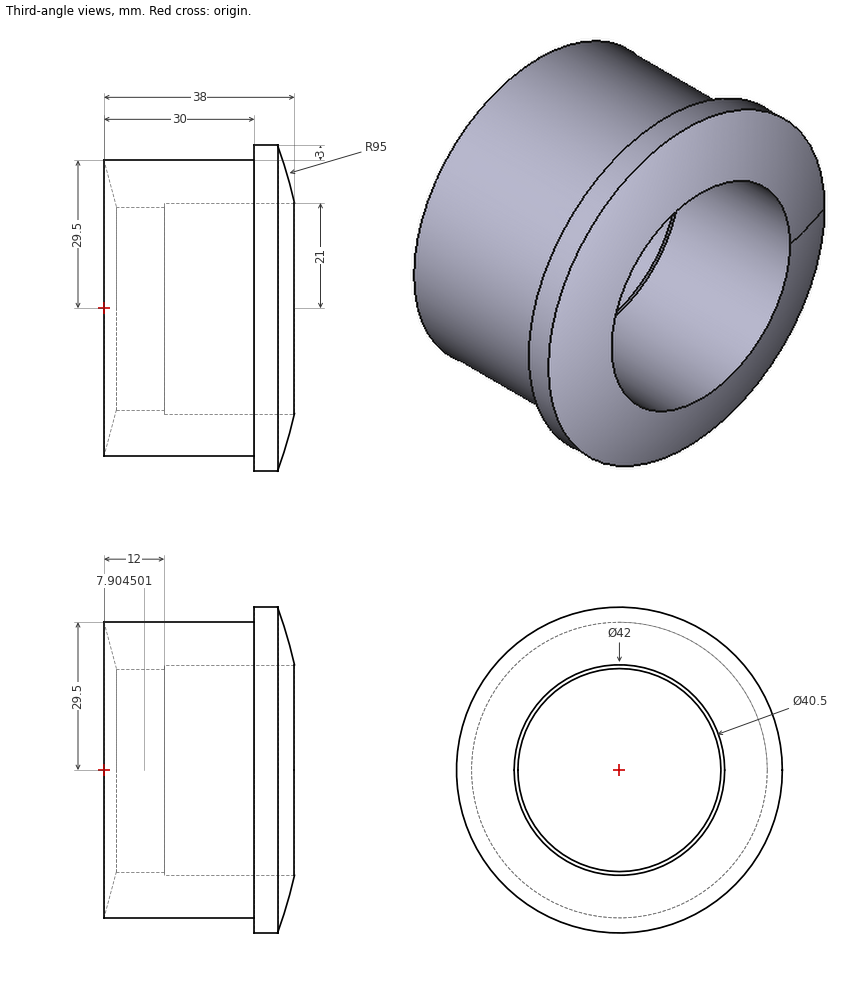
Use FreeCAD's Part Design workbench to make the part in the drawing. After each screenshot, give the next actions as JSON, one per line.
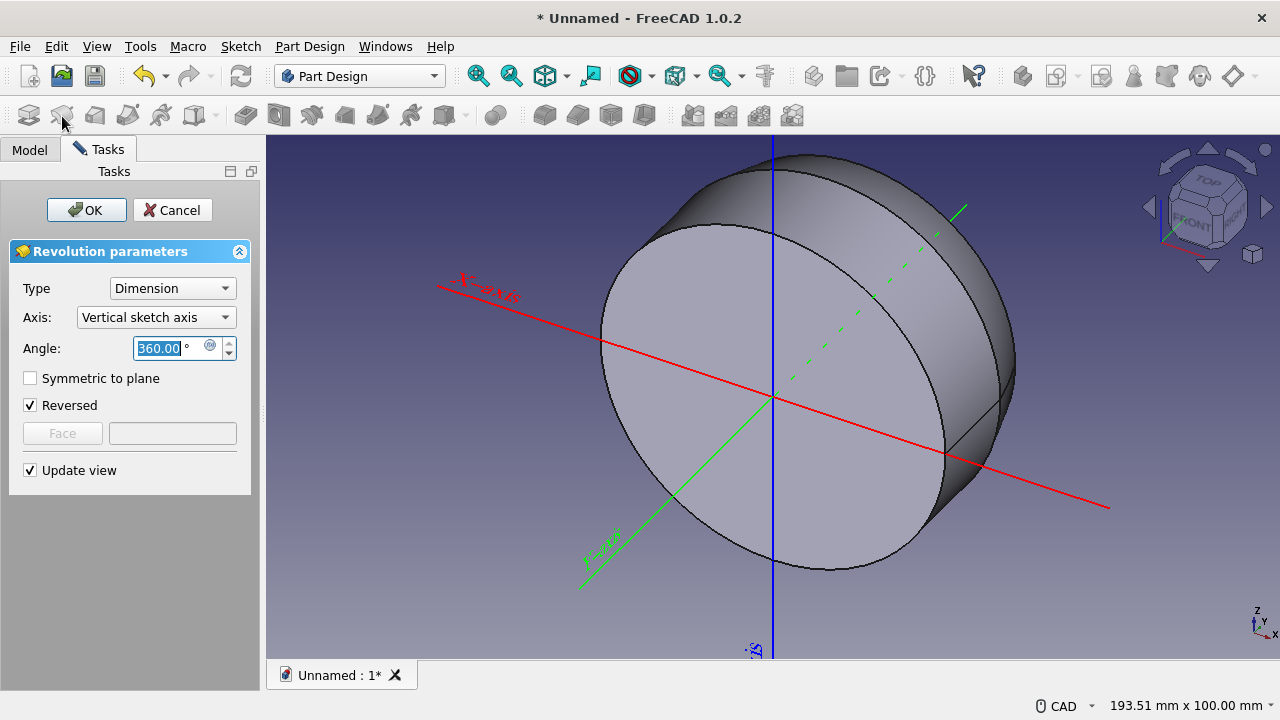
{"action": "left_click", "coordinate": [157, 318]}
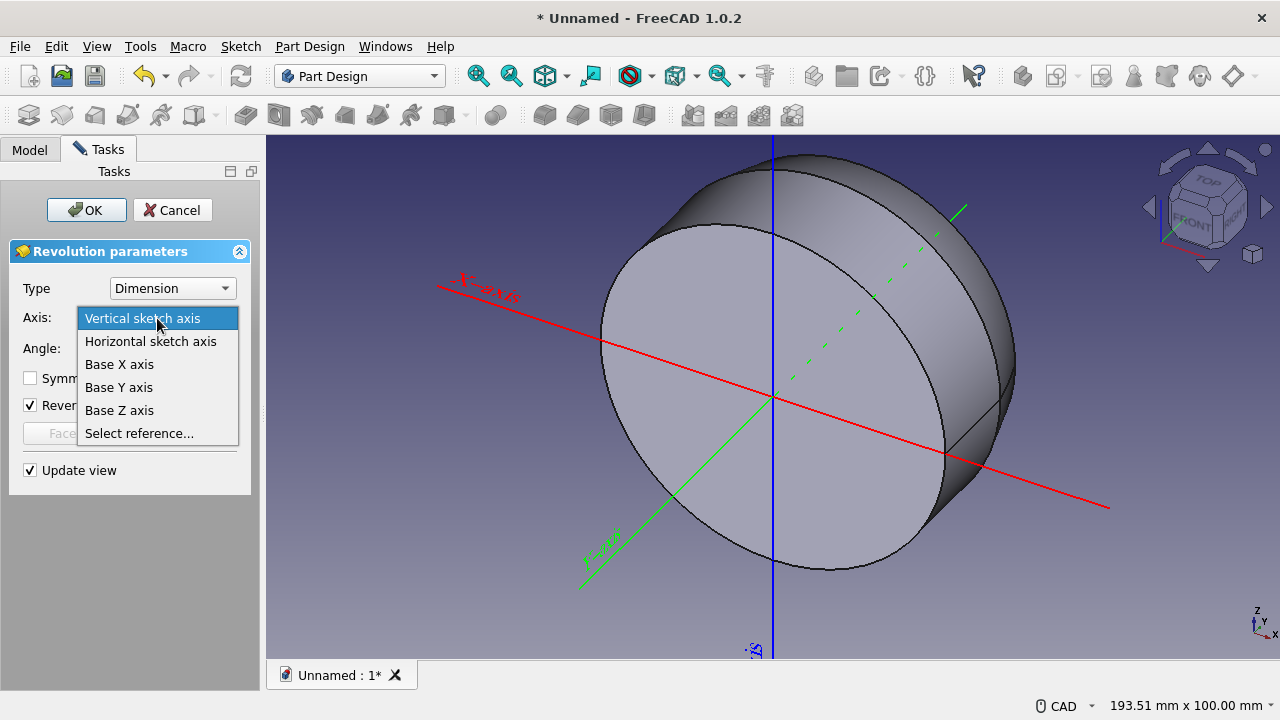
{"action": "left_click", "coordinate": [156, 342]}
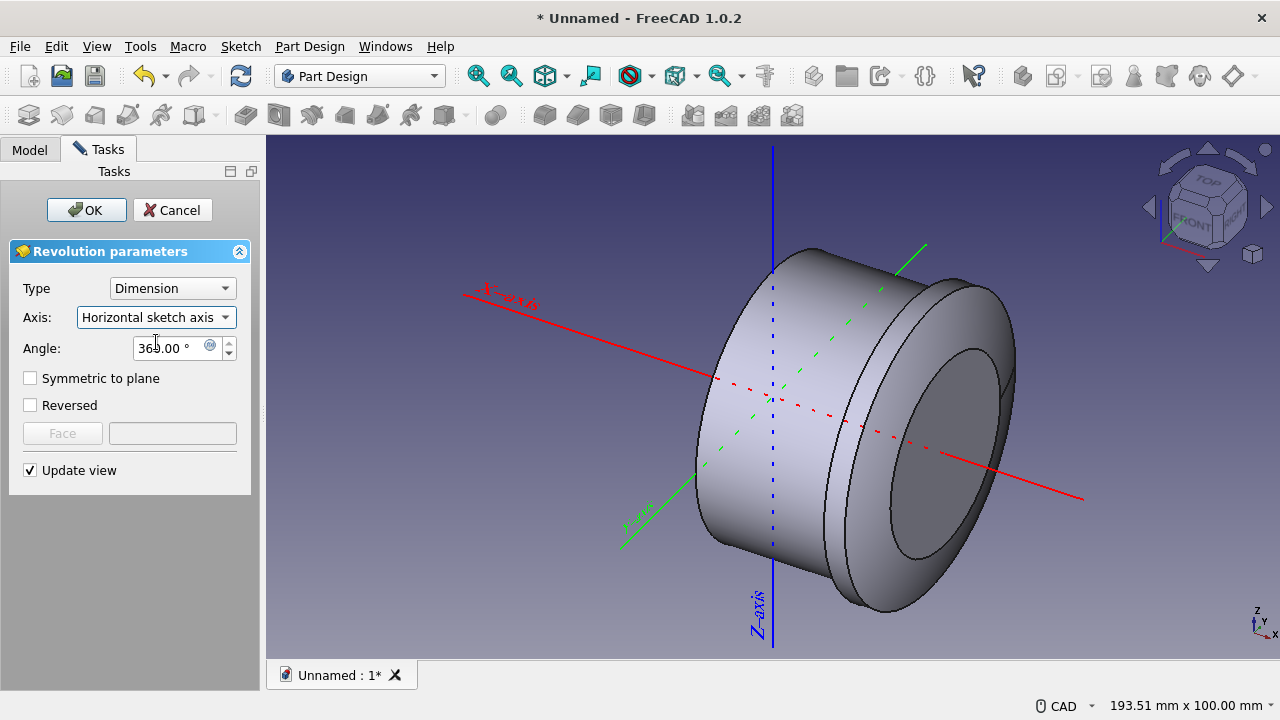
{"action": "left_click", "coordinate": [87, 210]}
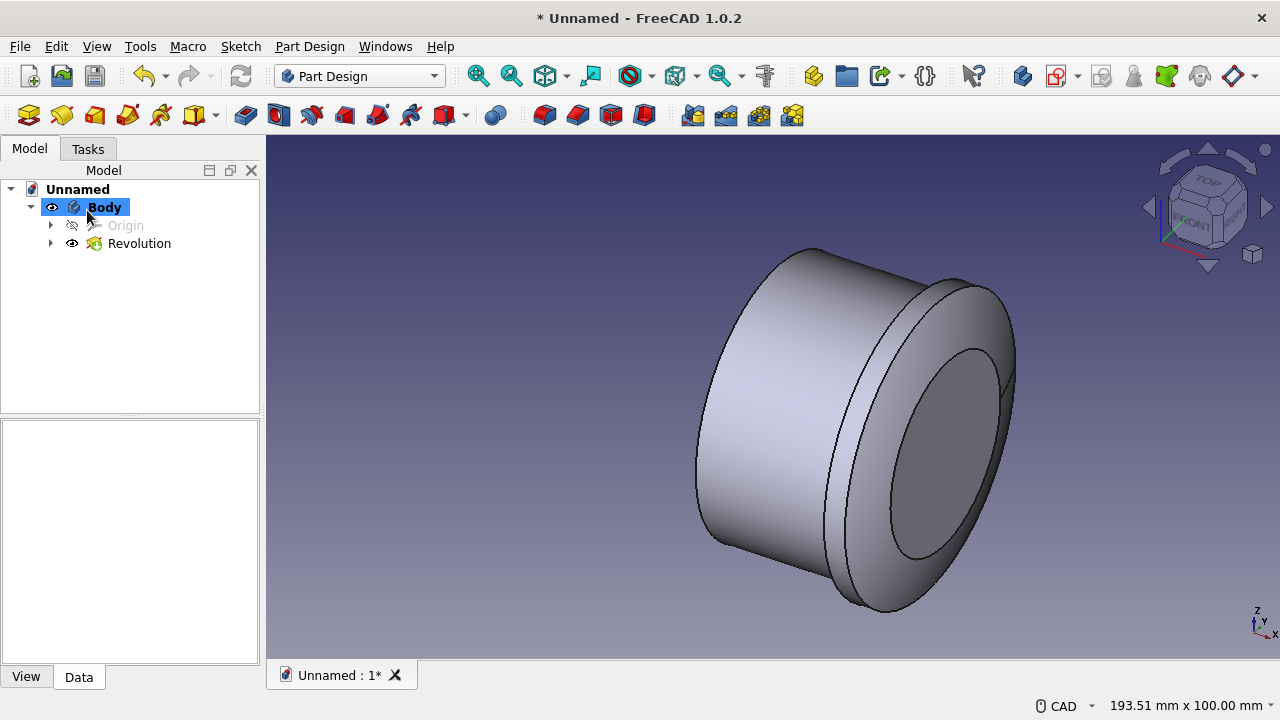
{"action": "left_click", "coordinate": [479, 76]}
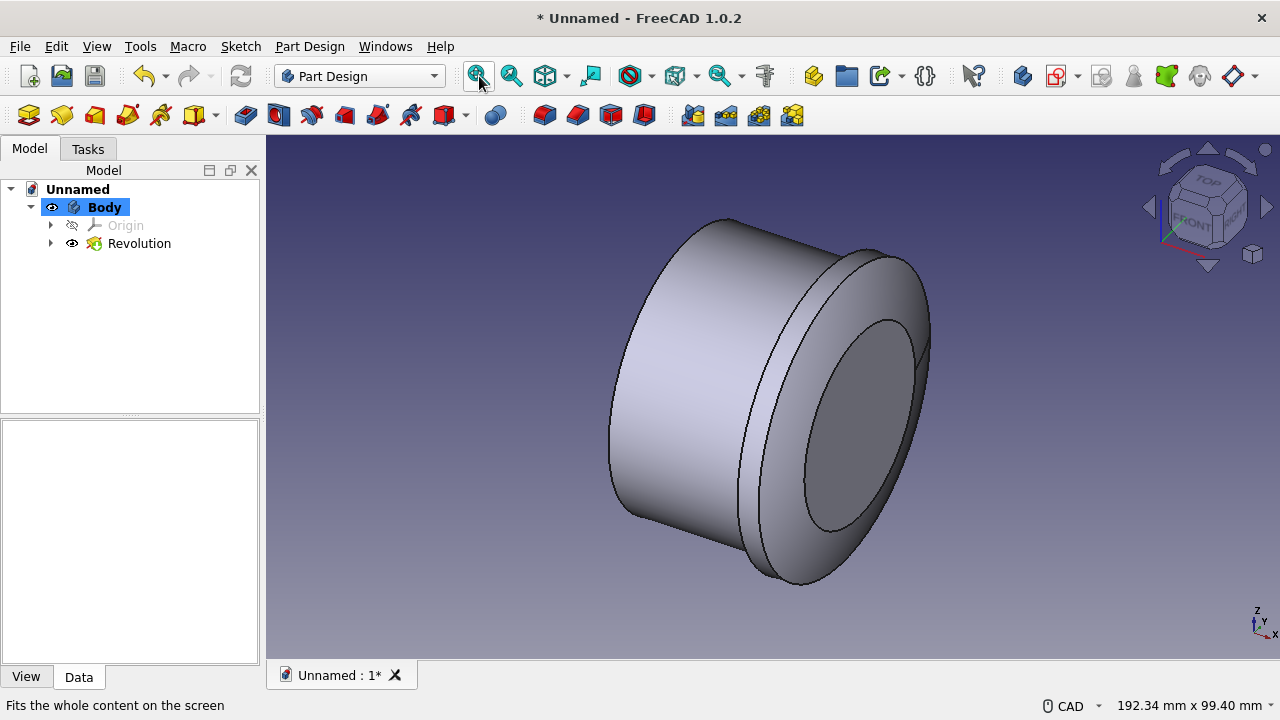
{"action": "key", "text": "6"}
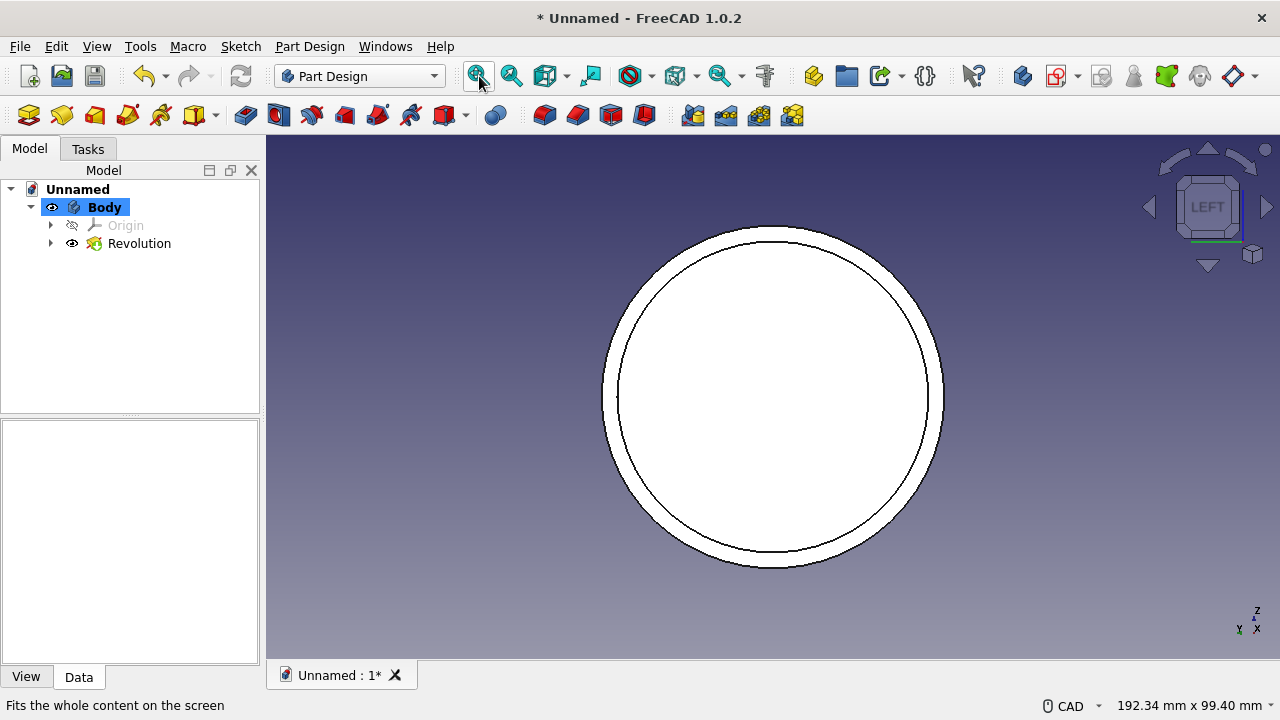
{"action": "left_click", "coordinate": [773, 396]}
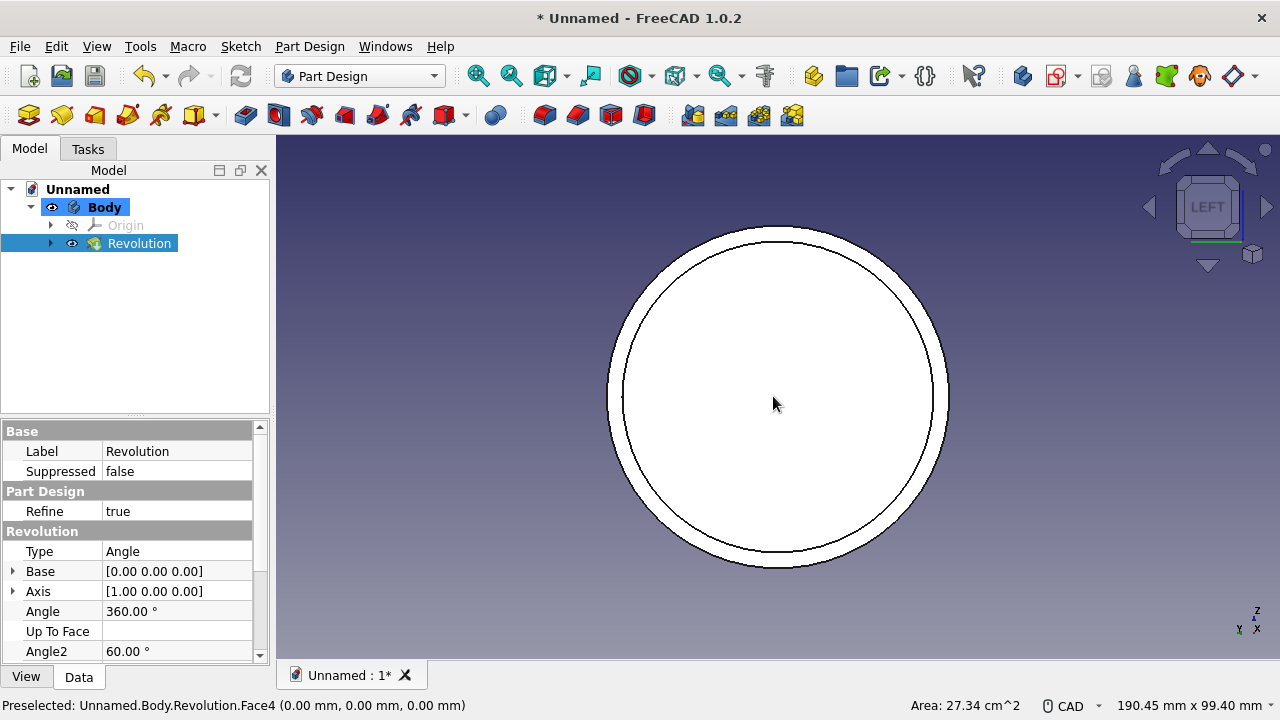
{"action": "left_click", "coordinate": [1056, 76]}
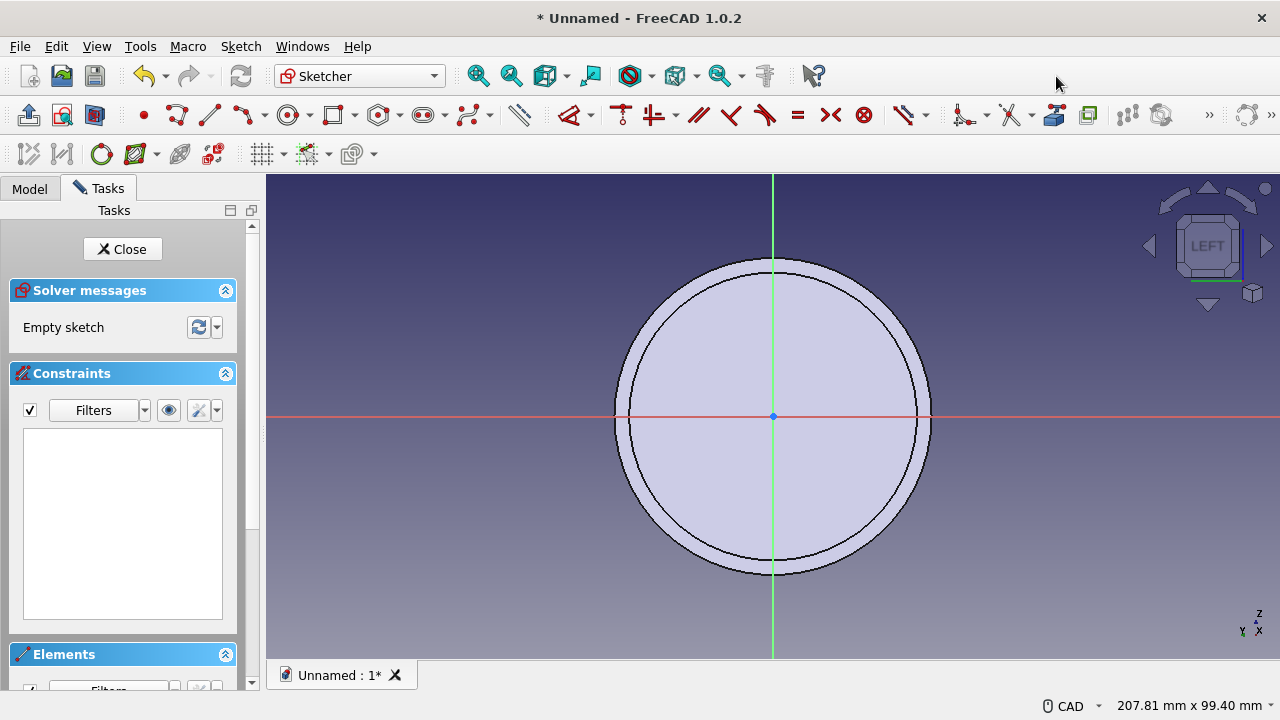
{"action": "scroll", "coordinate": [912, 416], "scroll_direction": "up", "scroll_amount": 2}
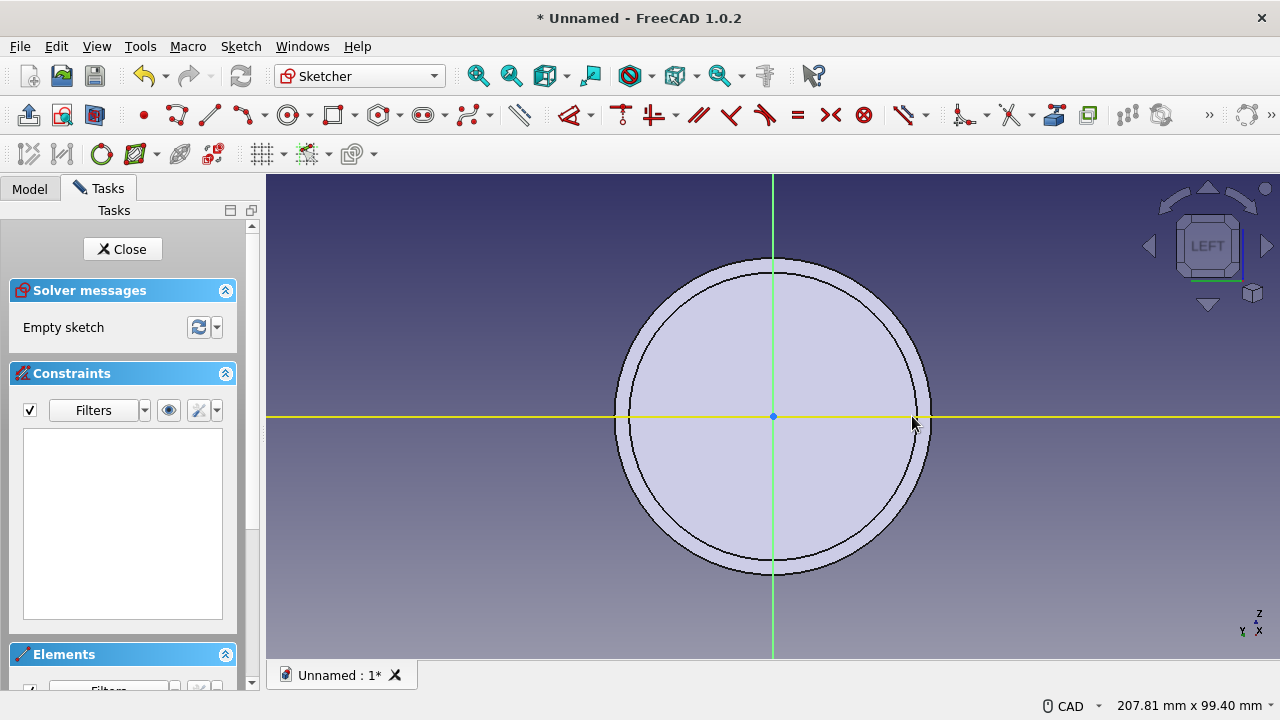
{"action": "left_click", "coordinate": [288, 116]}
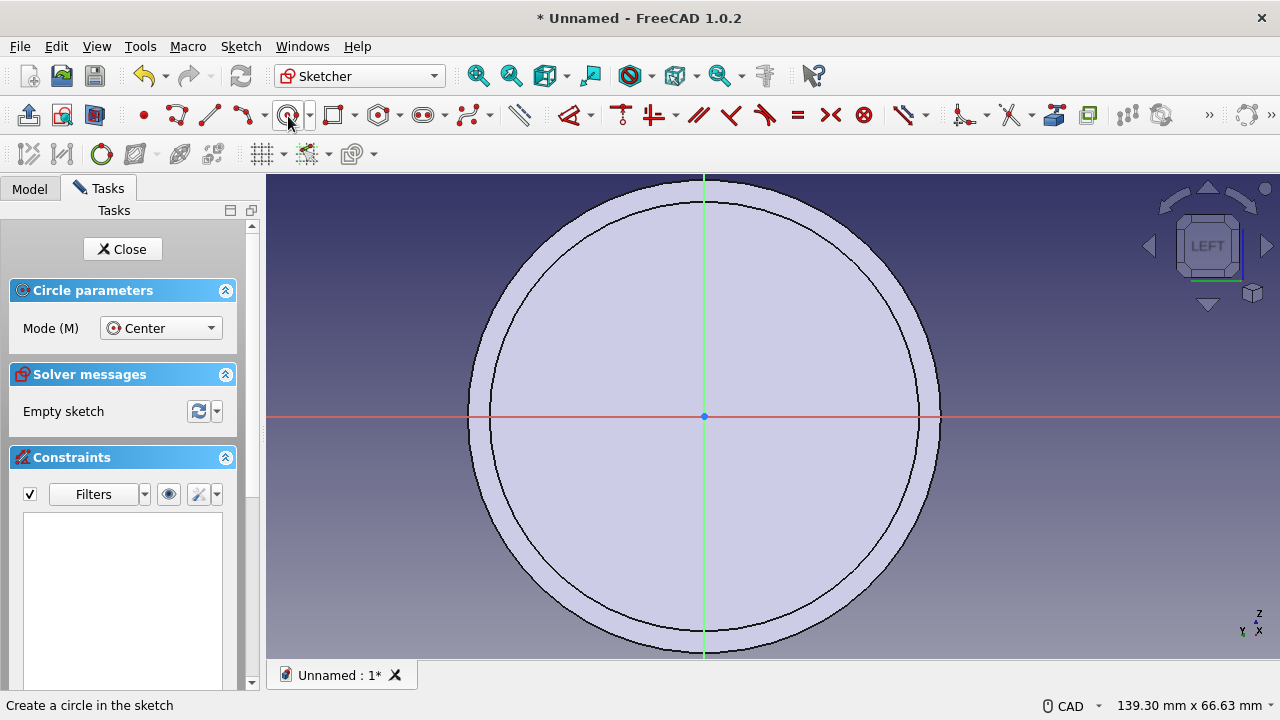
{"action": "left_click", "coordinate": [704, 416]}
{"action": "mouse_move", "coordinate": [809, 312]}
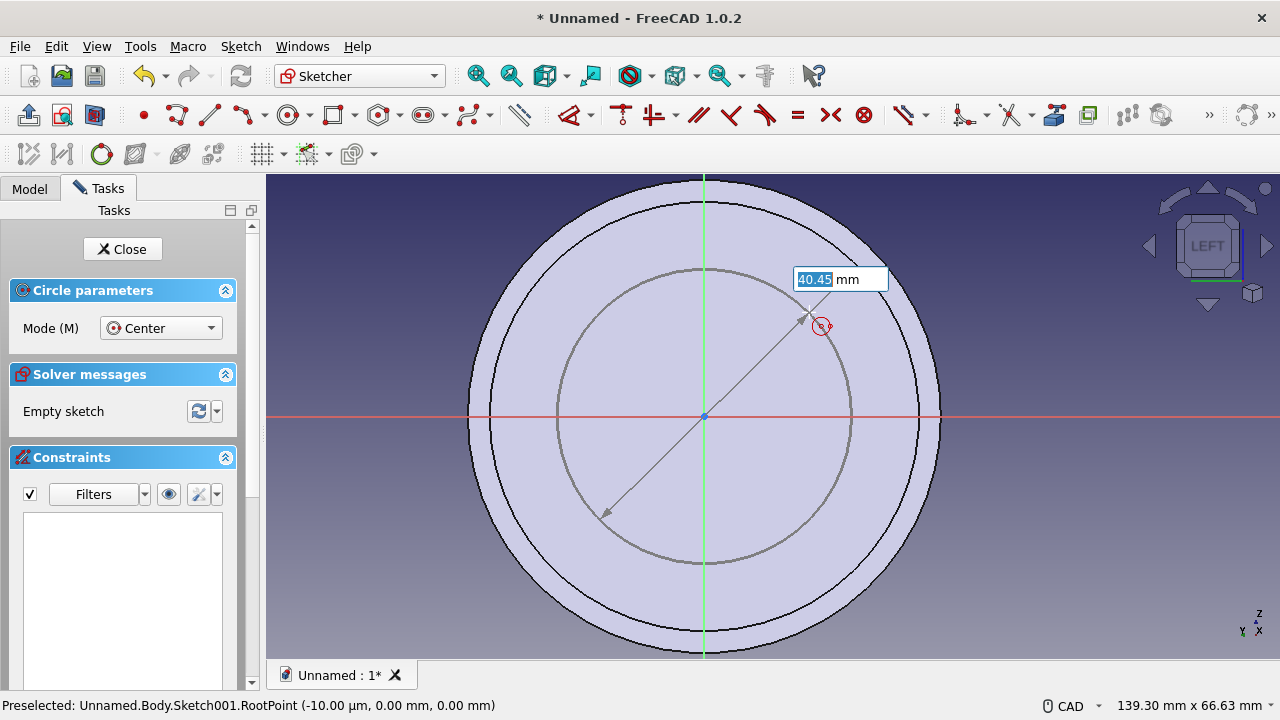
{"action": "type", "text": "40.5"}
{"action": "key", "text": "Return"}
{"action": "key", "text": "Escape"}